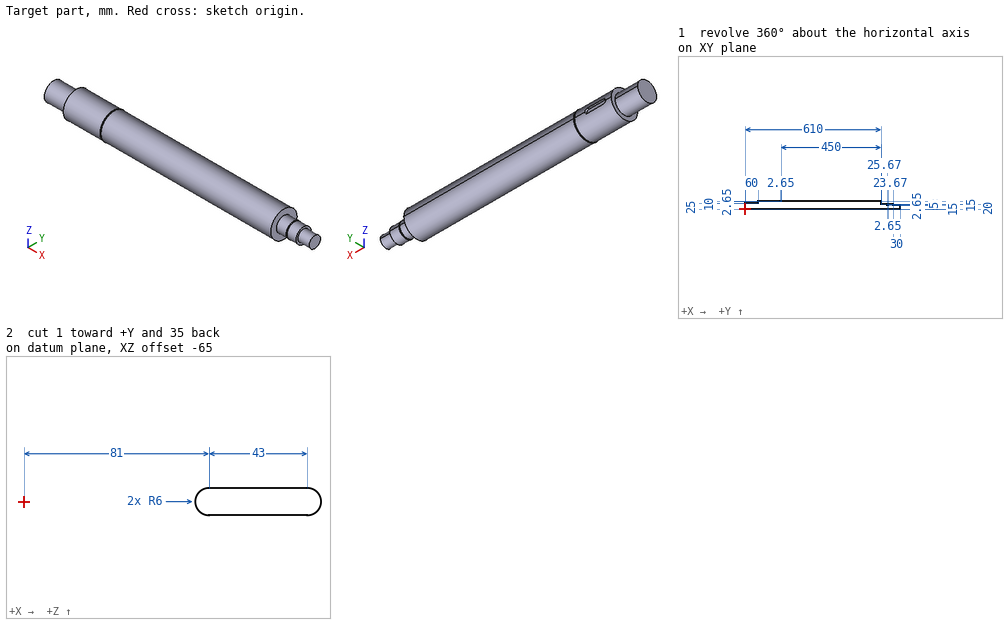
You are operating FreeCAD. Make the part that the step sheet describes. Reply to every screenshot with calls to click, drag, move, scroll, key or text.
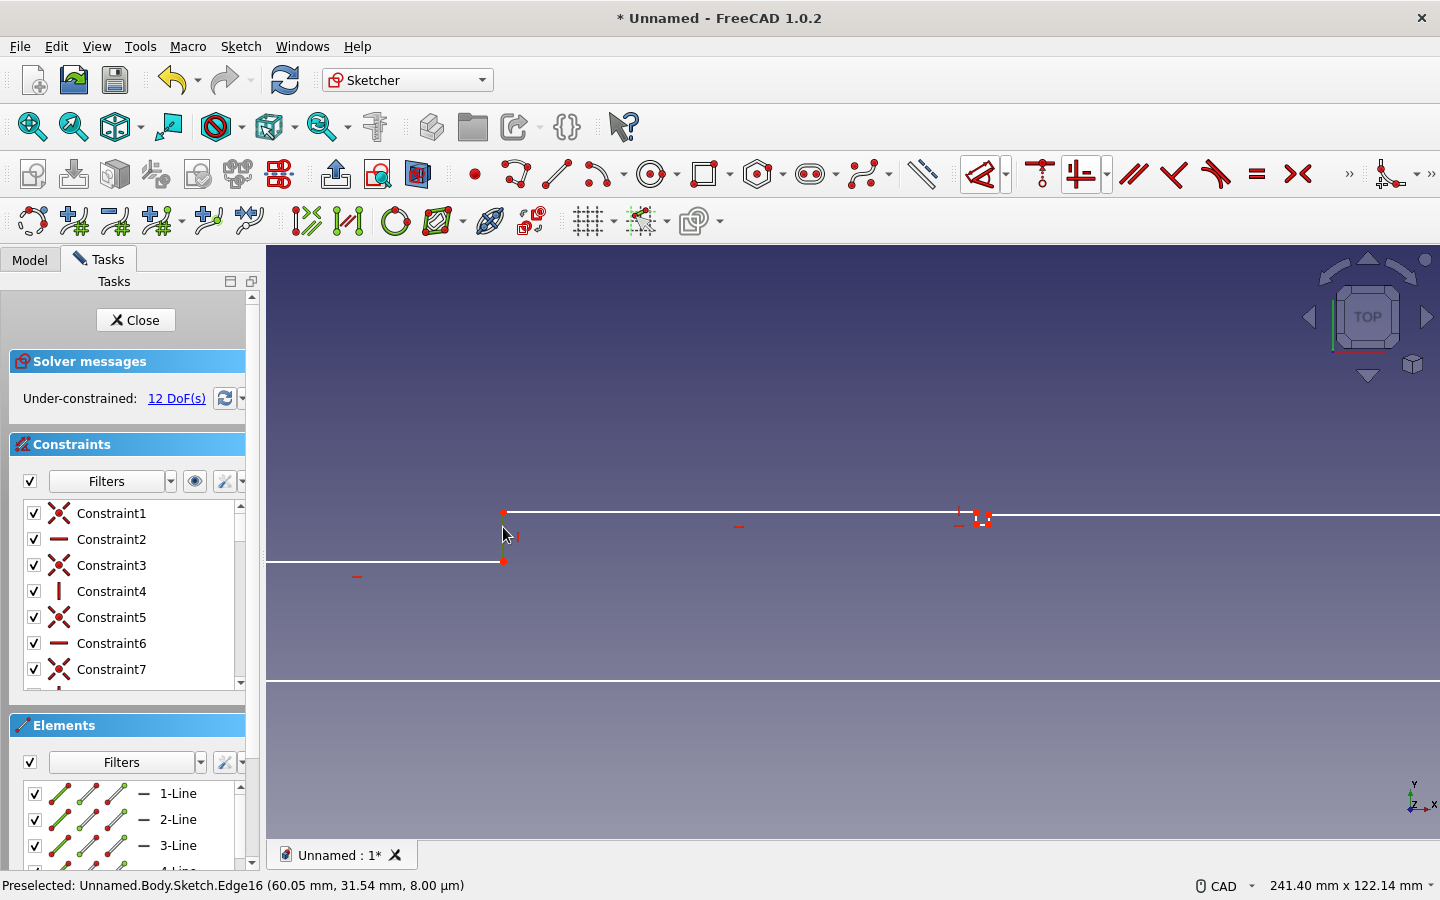
key(i)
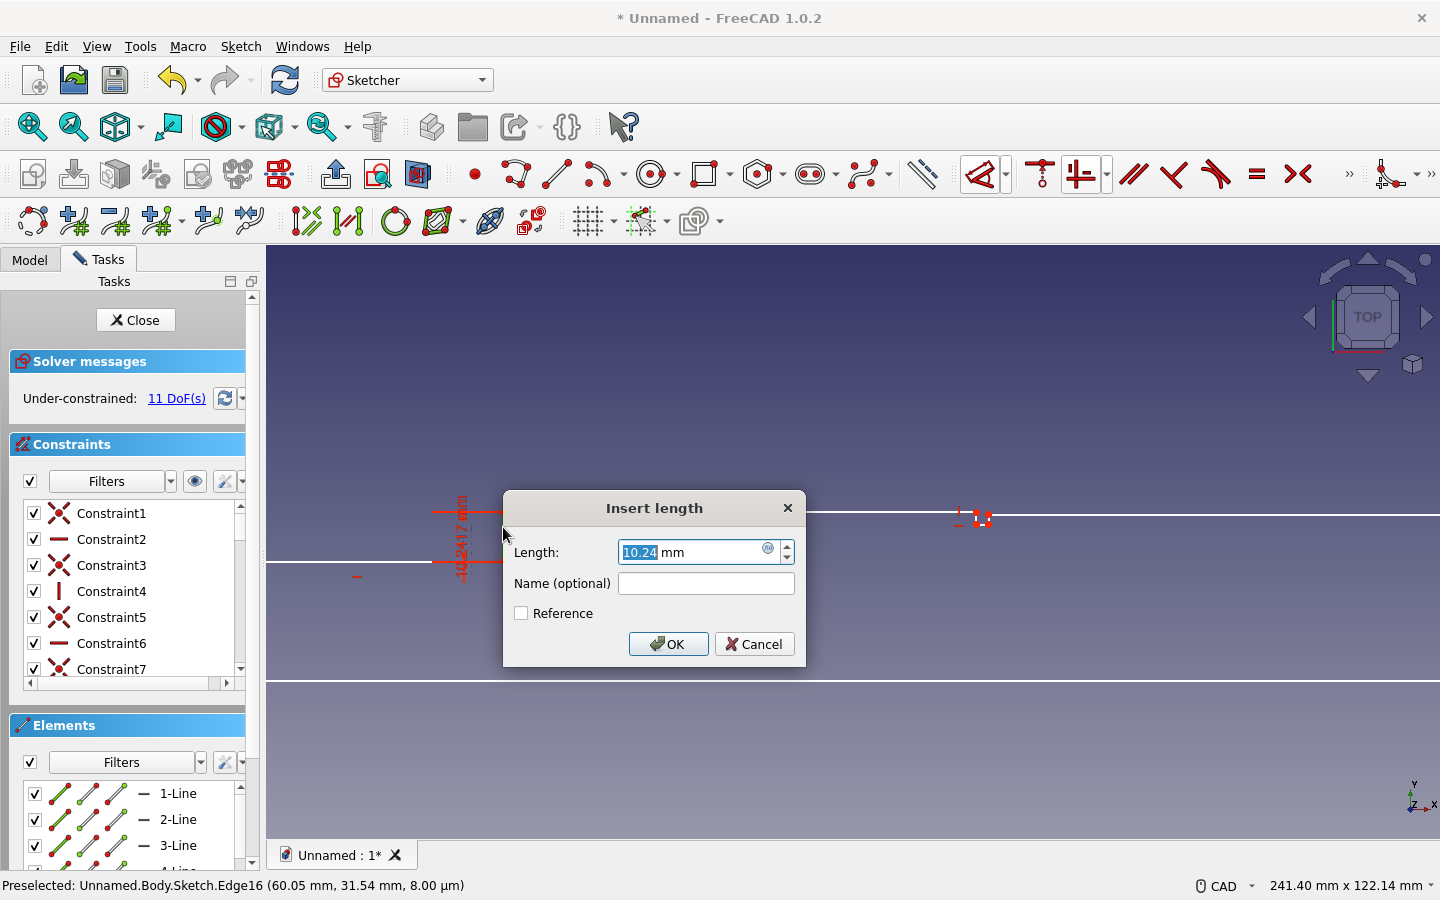
text(10)
key(Return)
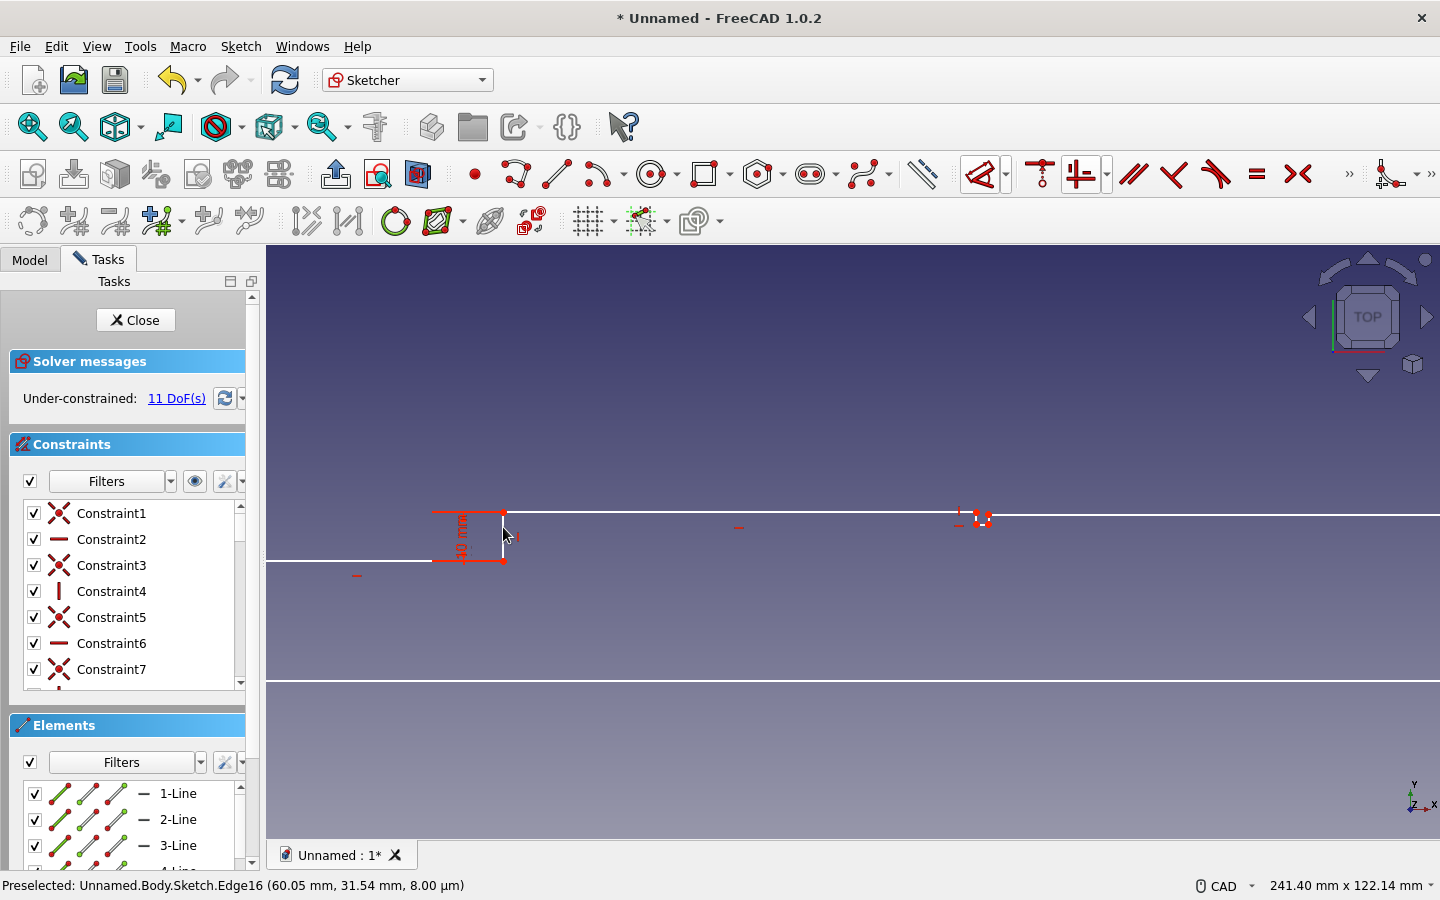
scroll(504, 528, down, 8)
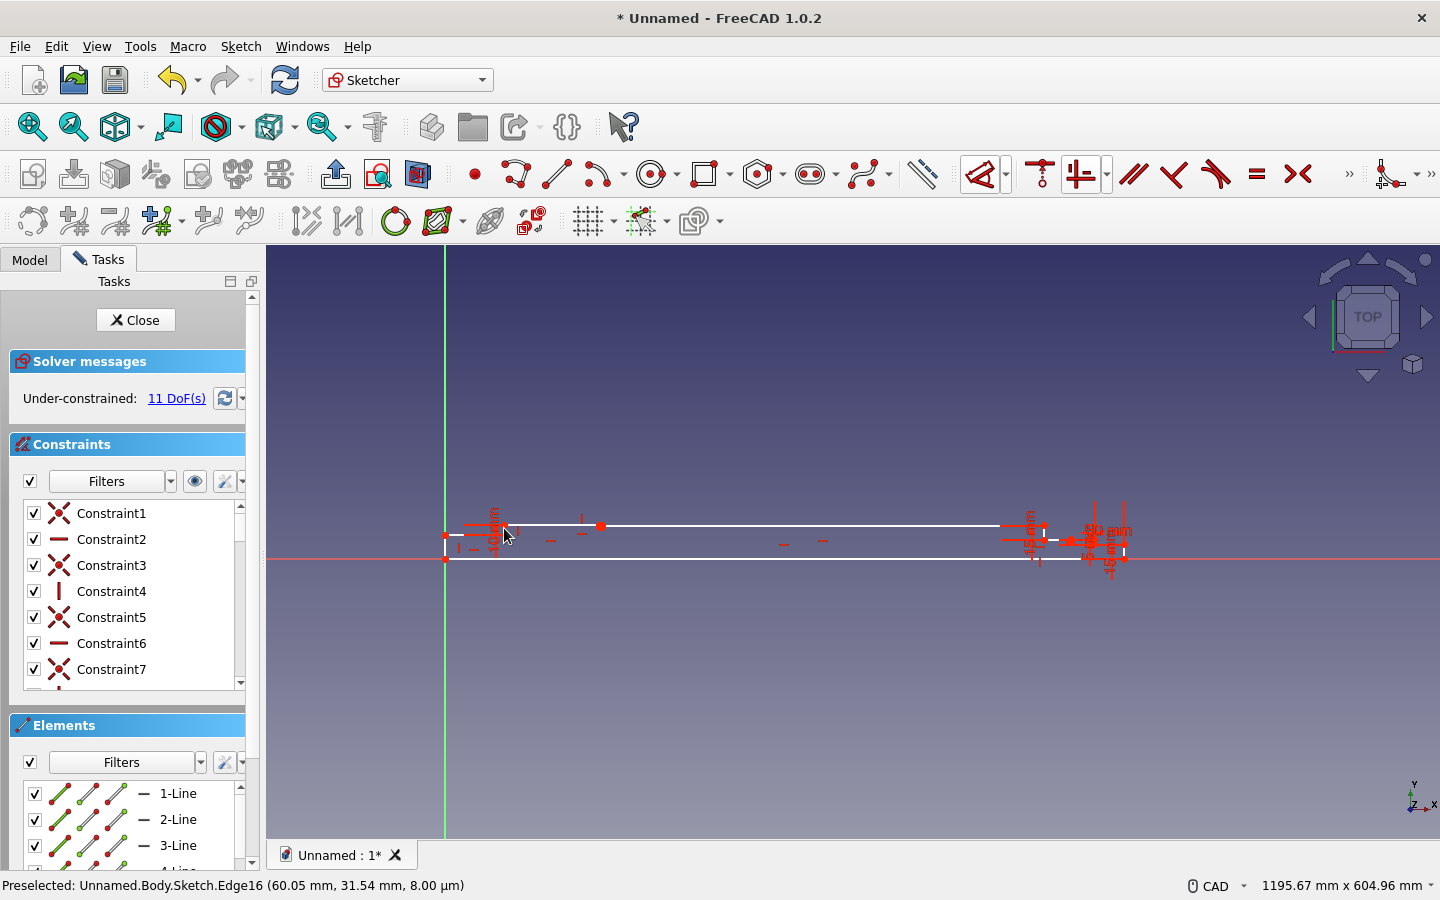
click(486, 535)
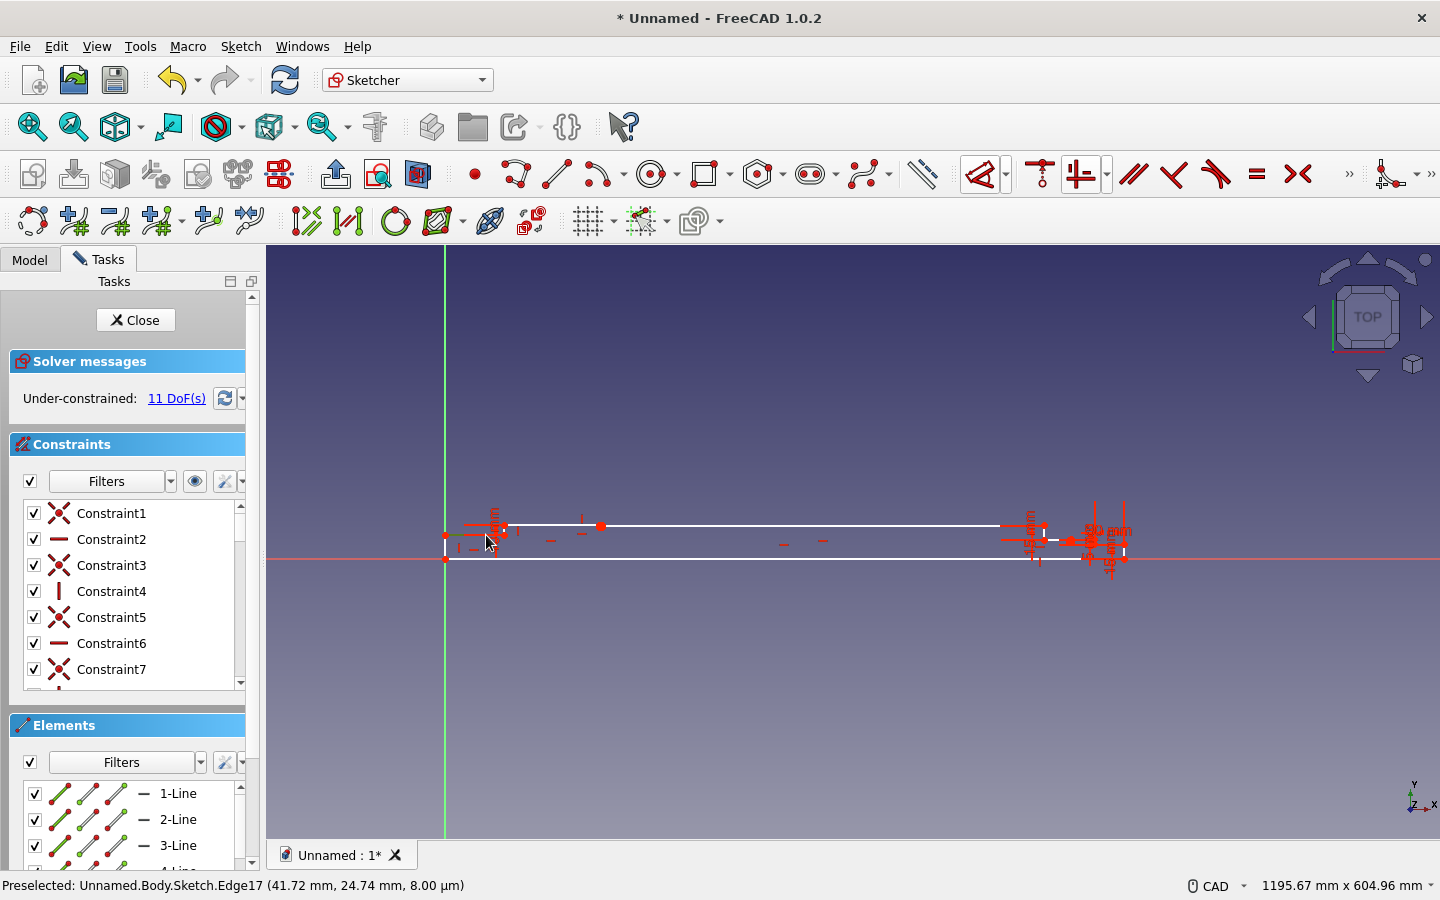
key(l)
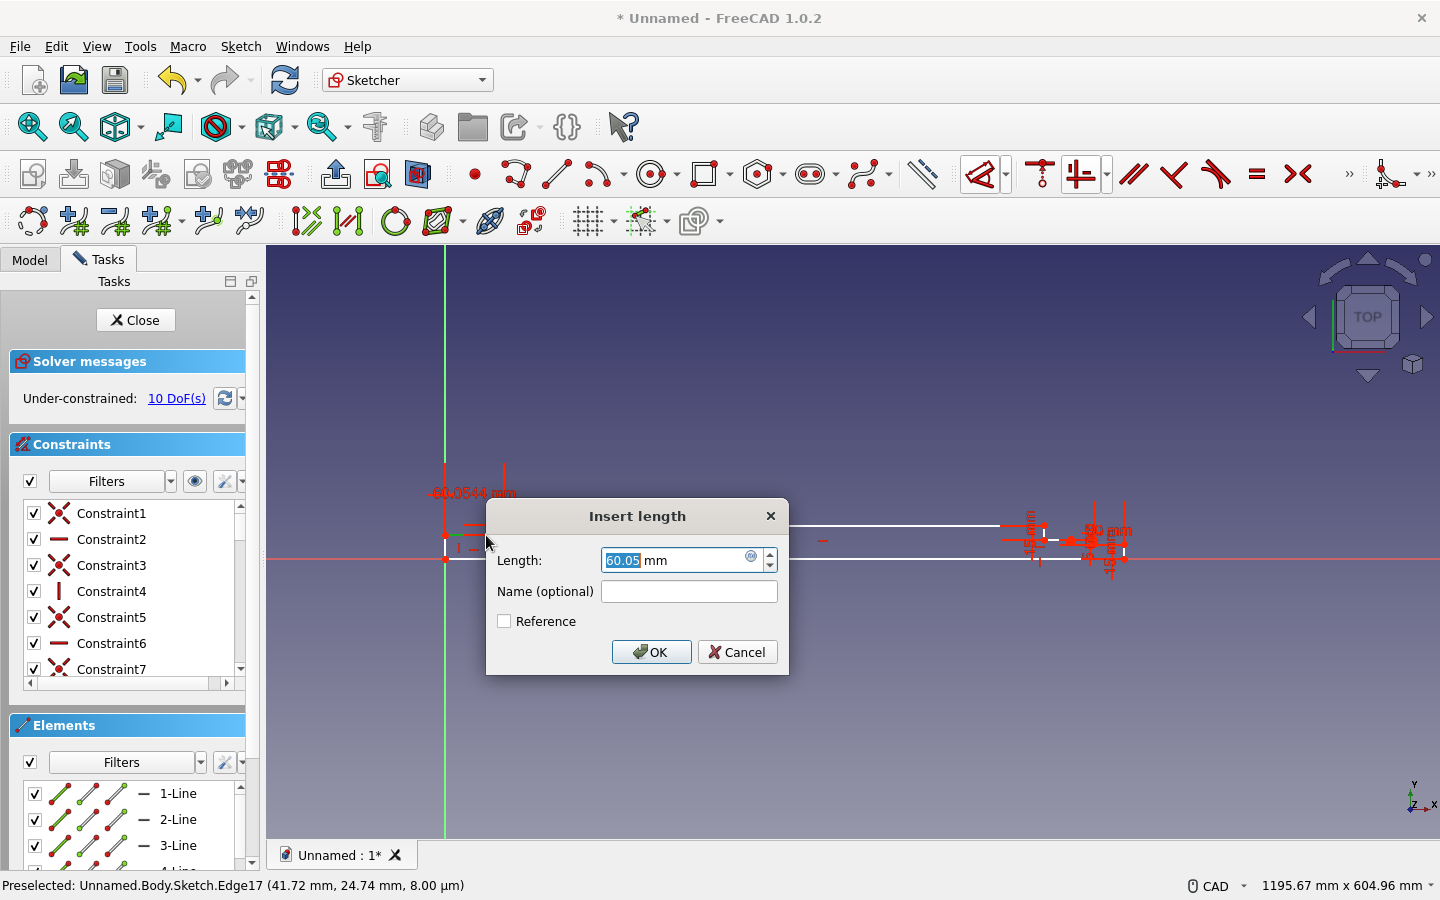
text(60)
key(Return)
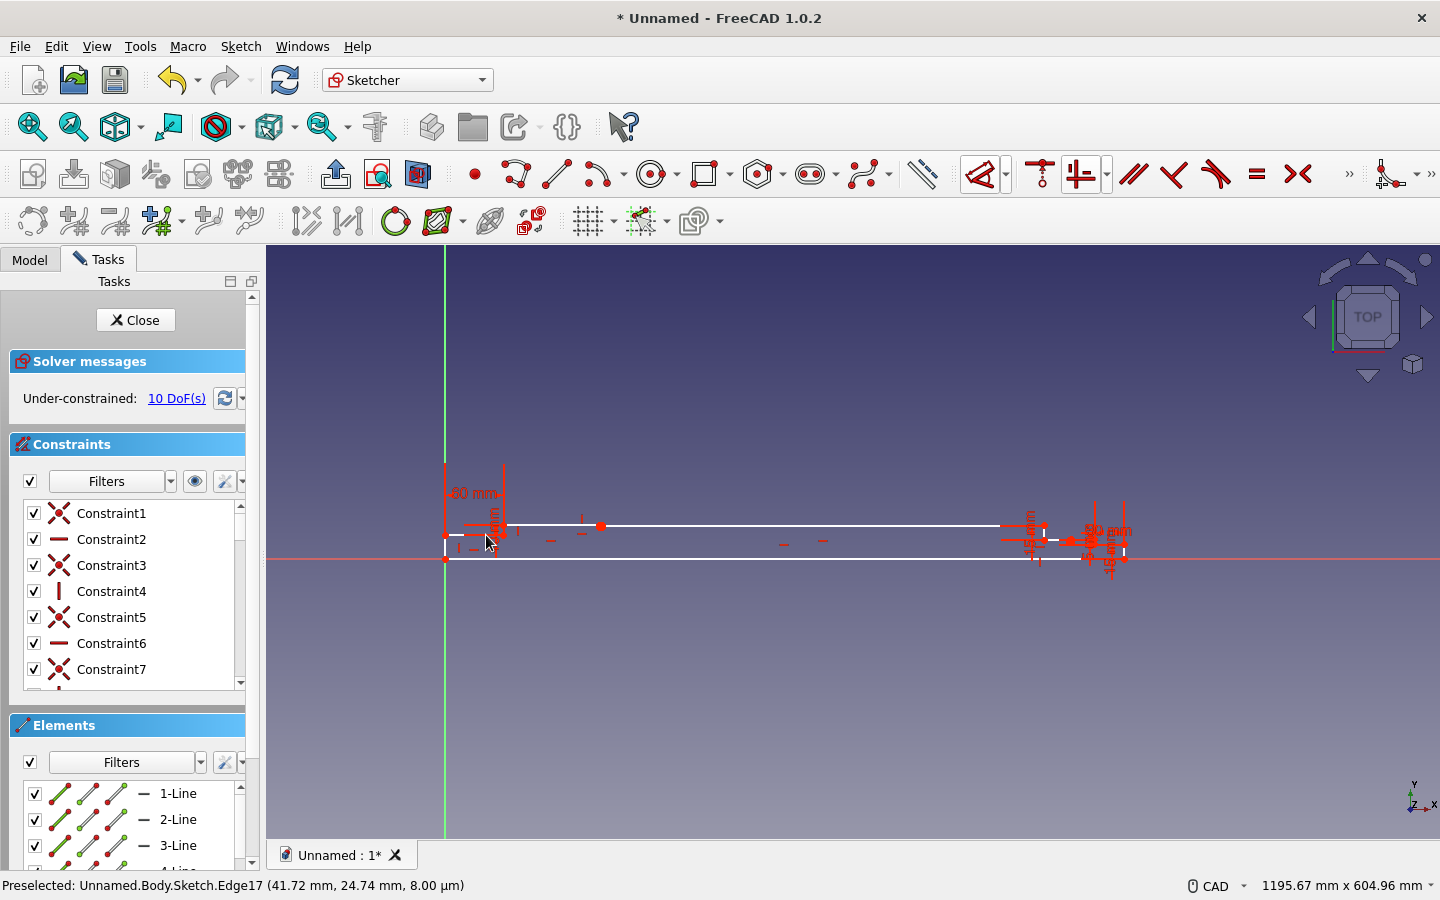
scroll(445, 545, up, 3)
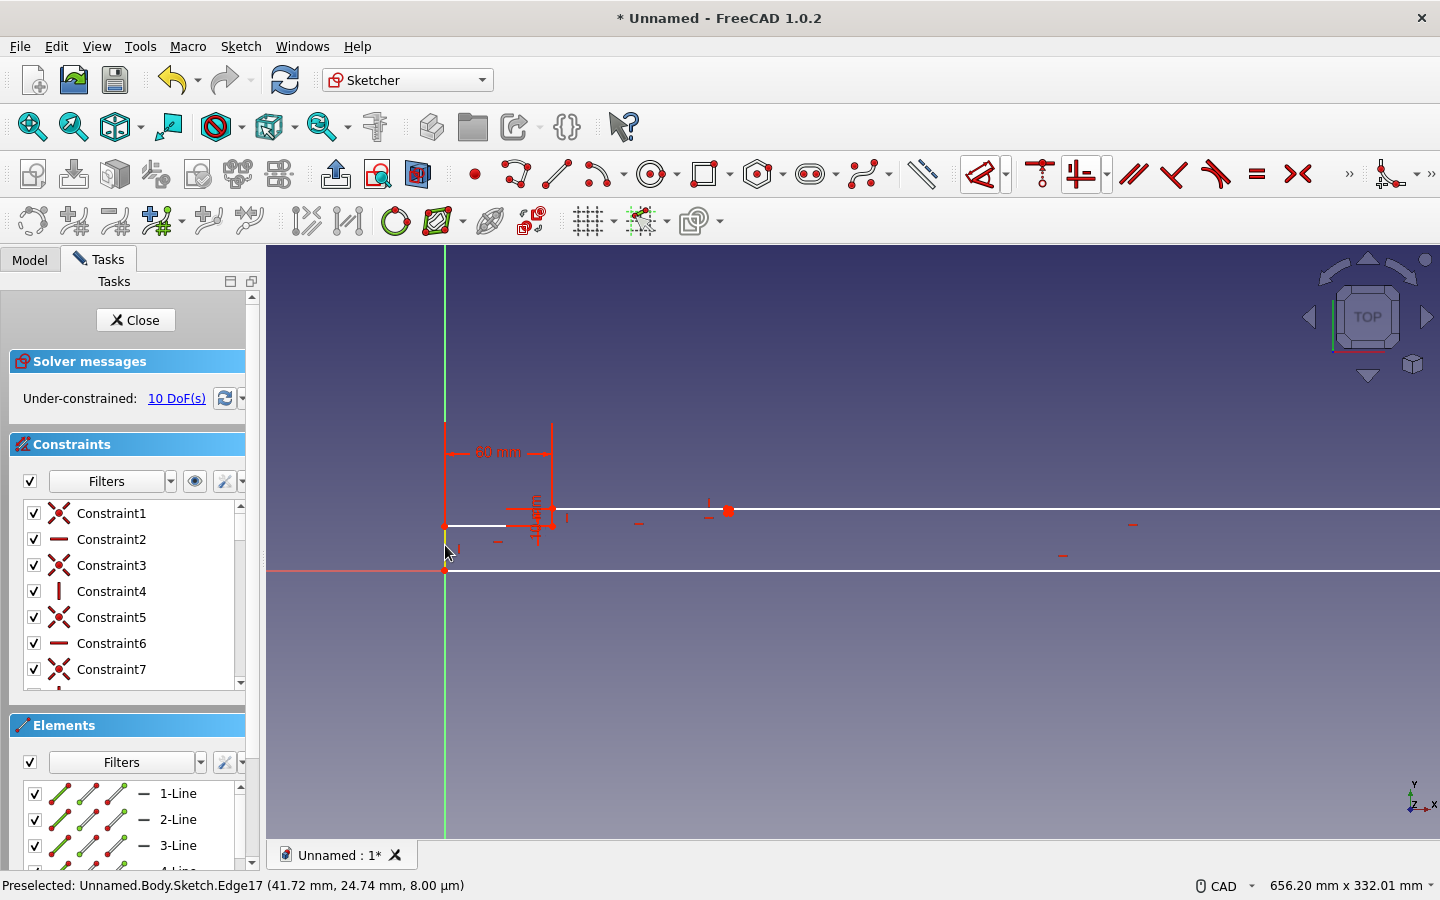
click(445, 544)